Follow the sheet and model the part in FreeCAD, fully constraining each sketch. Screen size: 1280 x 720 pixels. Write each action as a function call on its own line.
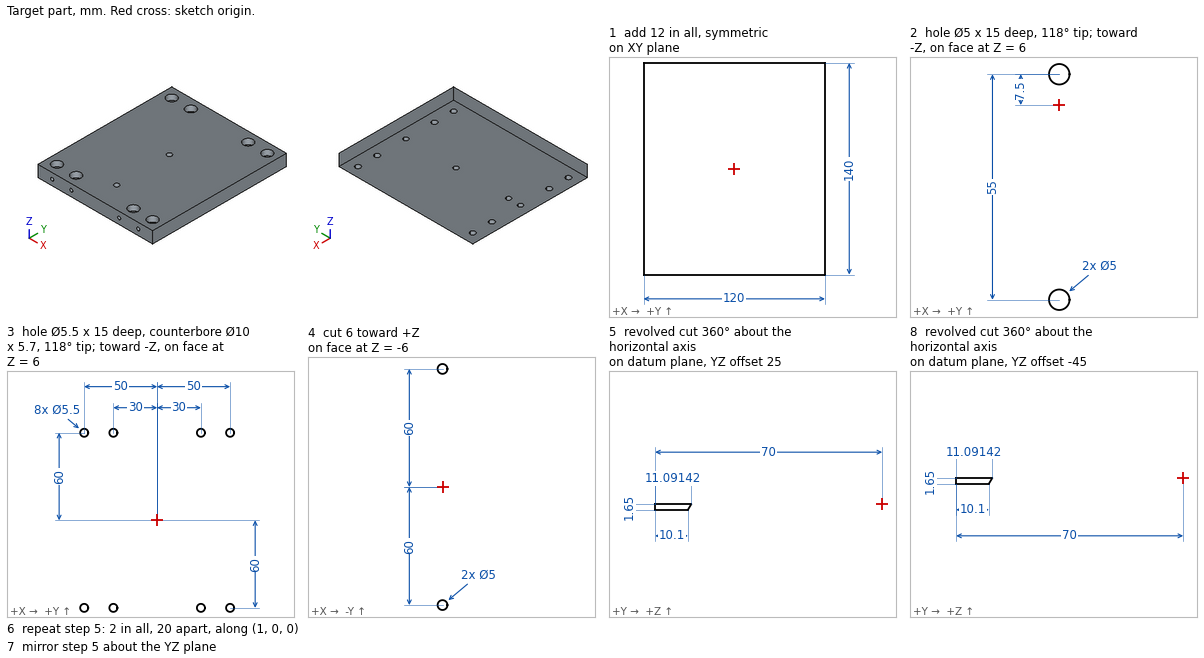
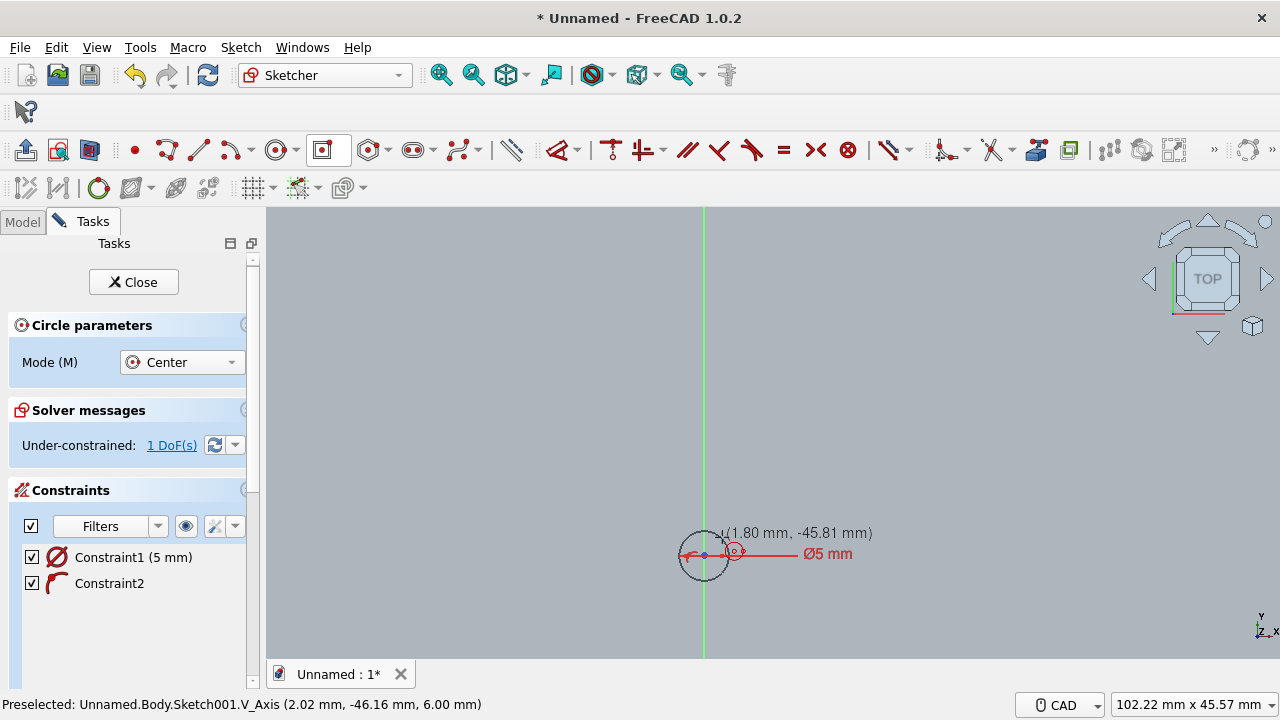
scroll(705, 556, down, 4)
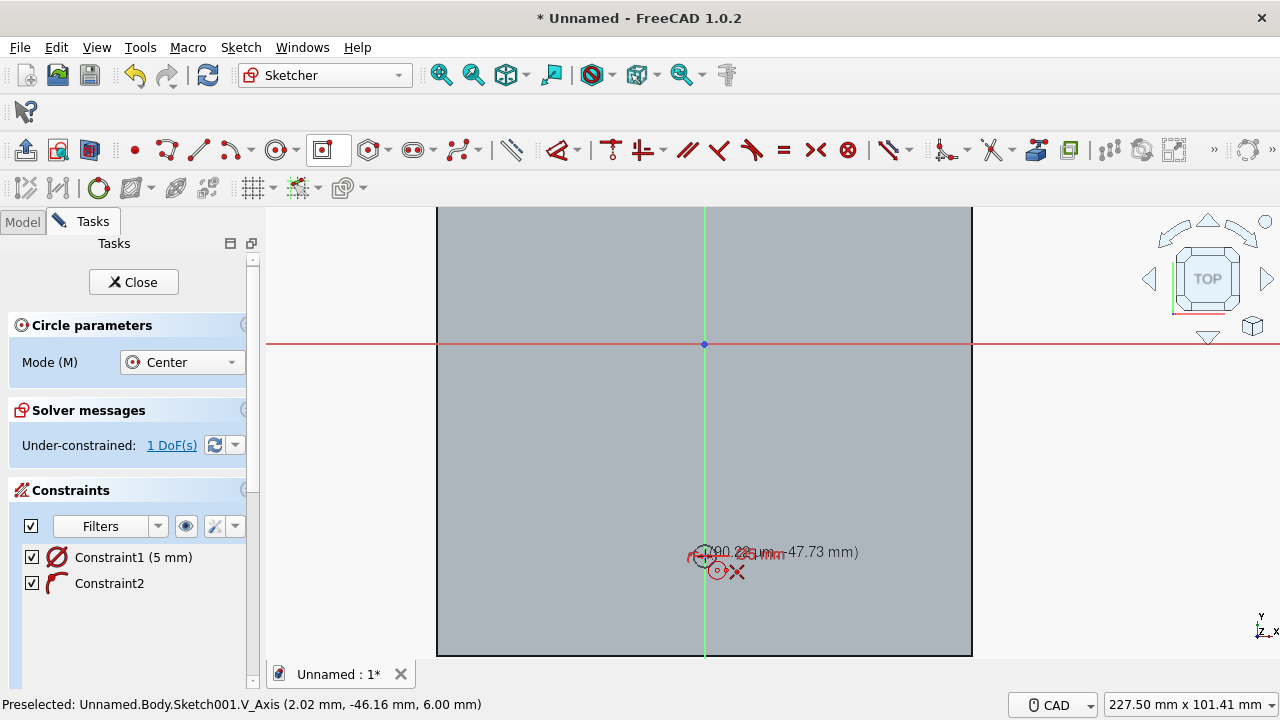
scroll(705, 311, up, 4)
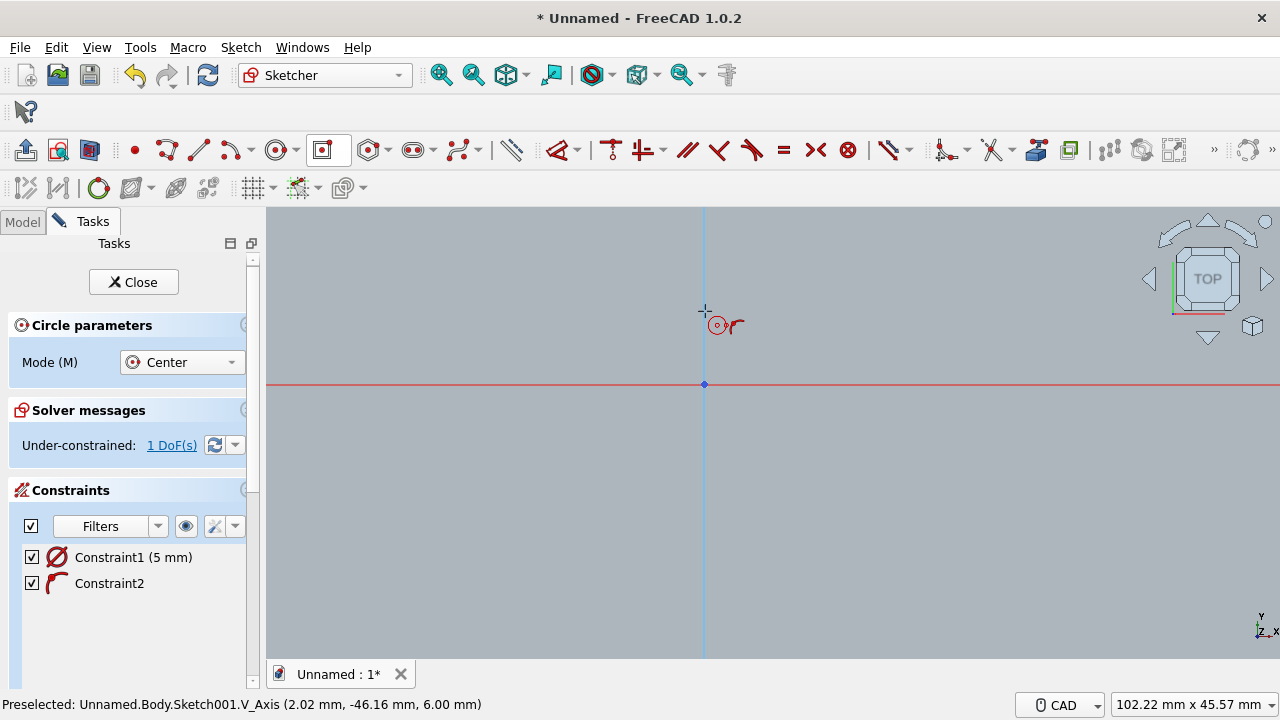
click(704, 310)
move(722, 293)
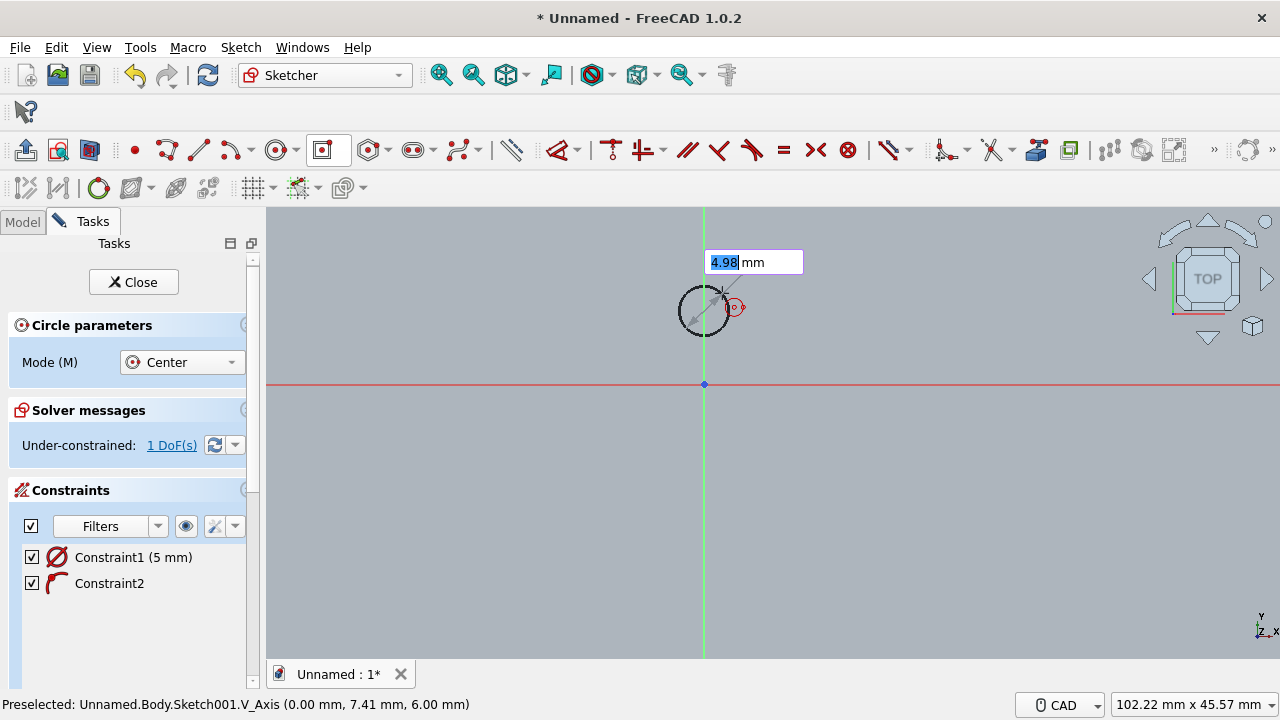
text(5)
key(Return)
key(Escape)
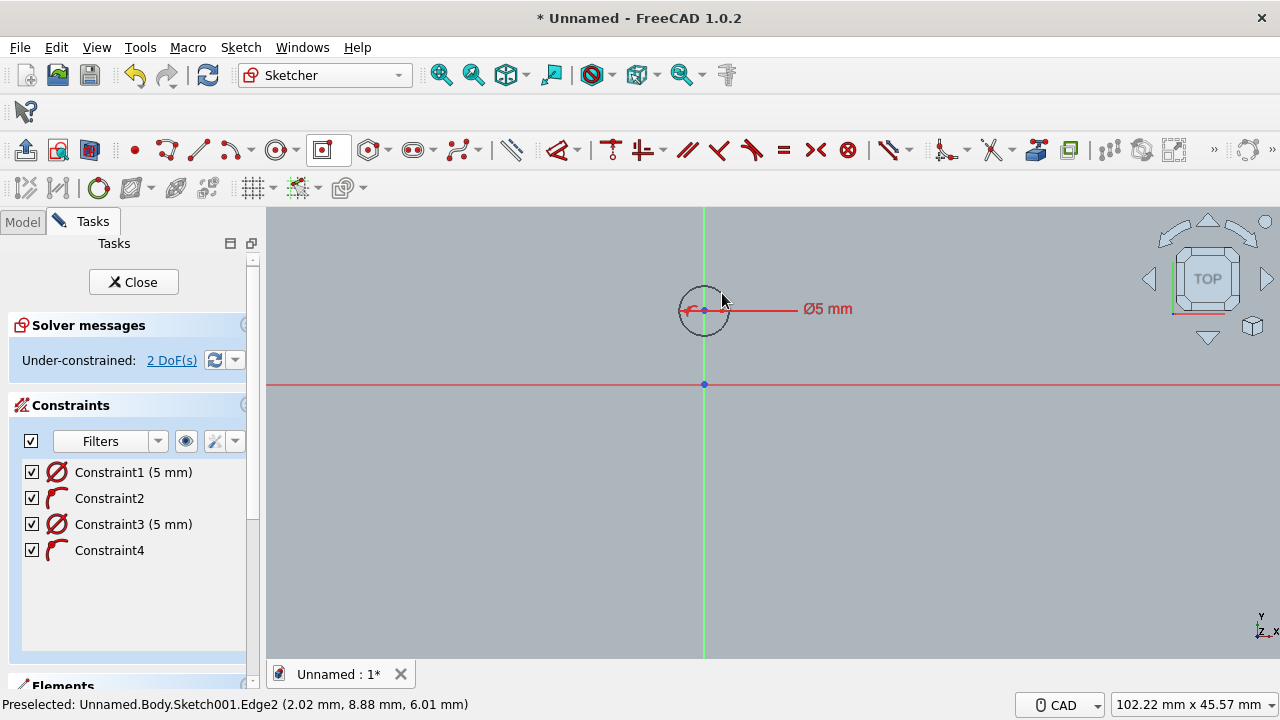
key(d)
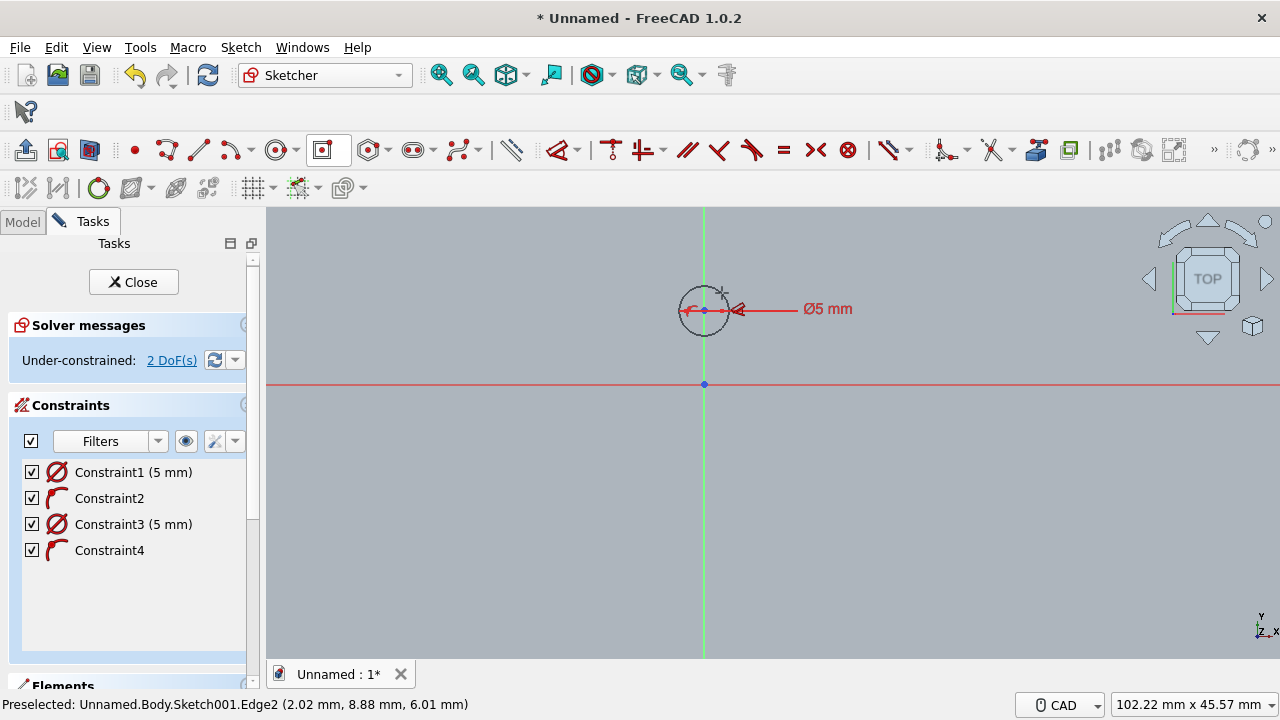
click(704, 311)
click(738, 348)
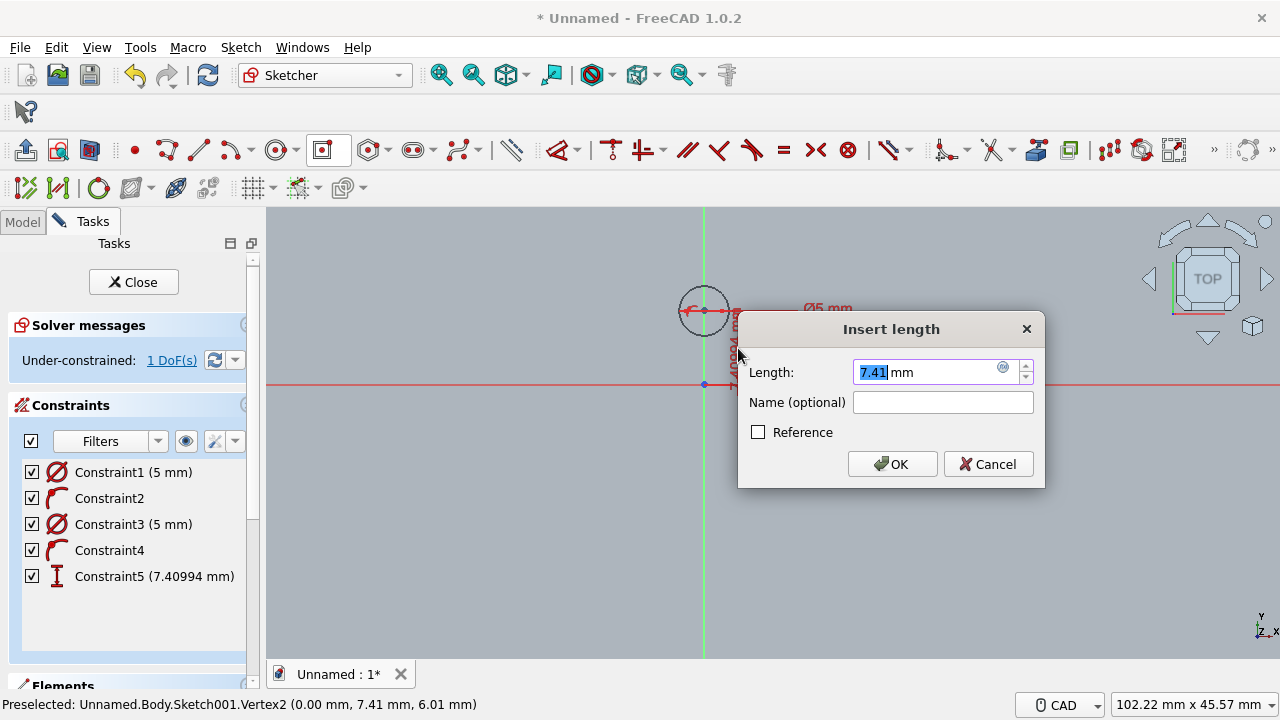
text(7.5)
key(Return)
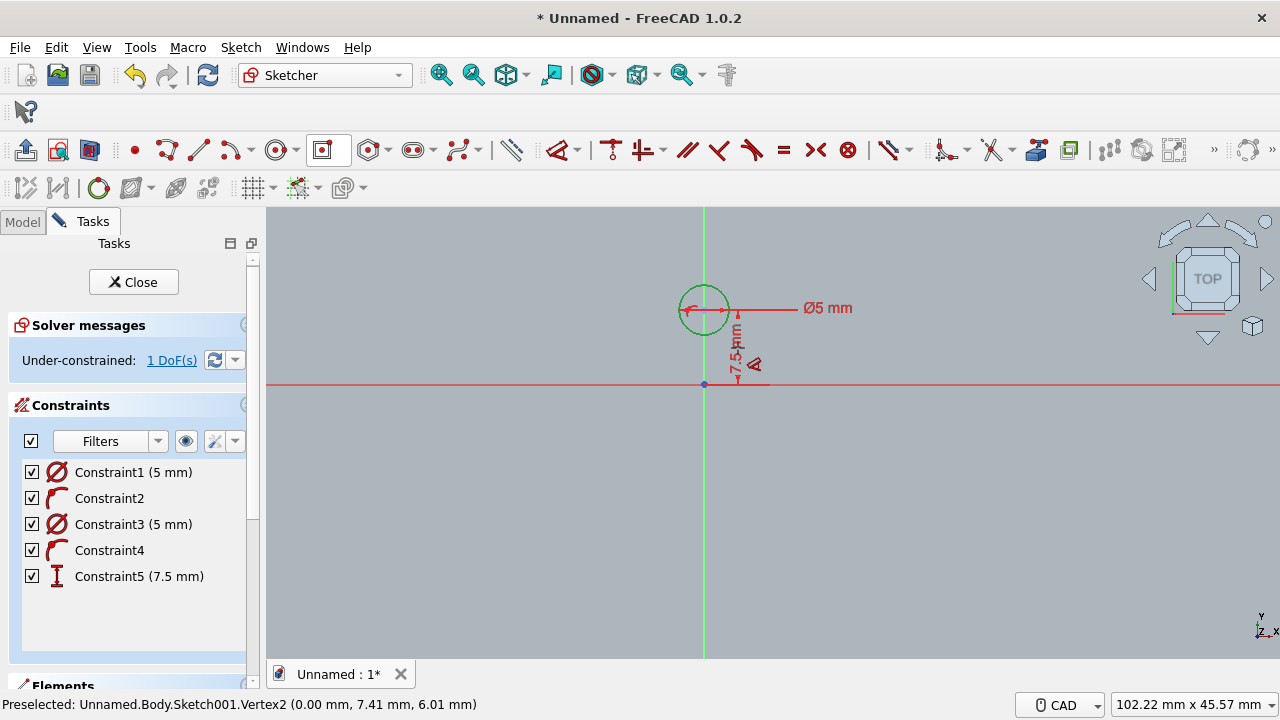
scroll(705, 311, down, 4)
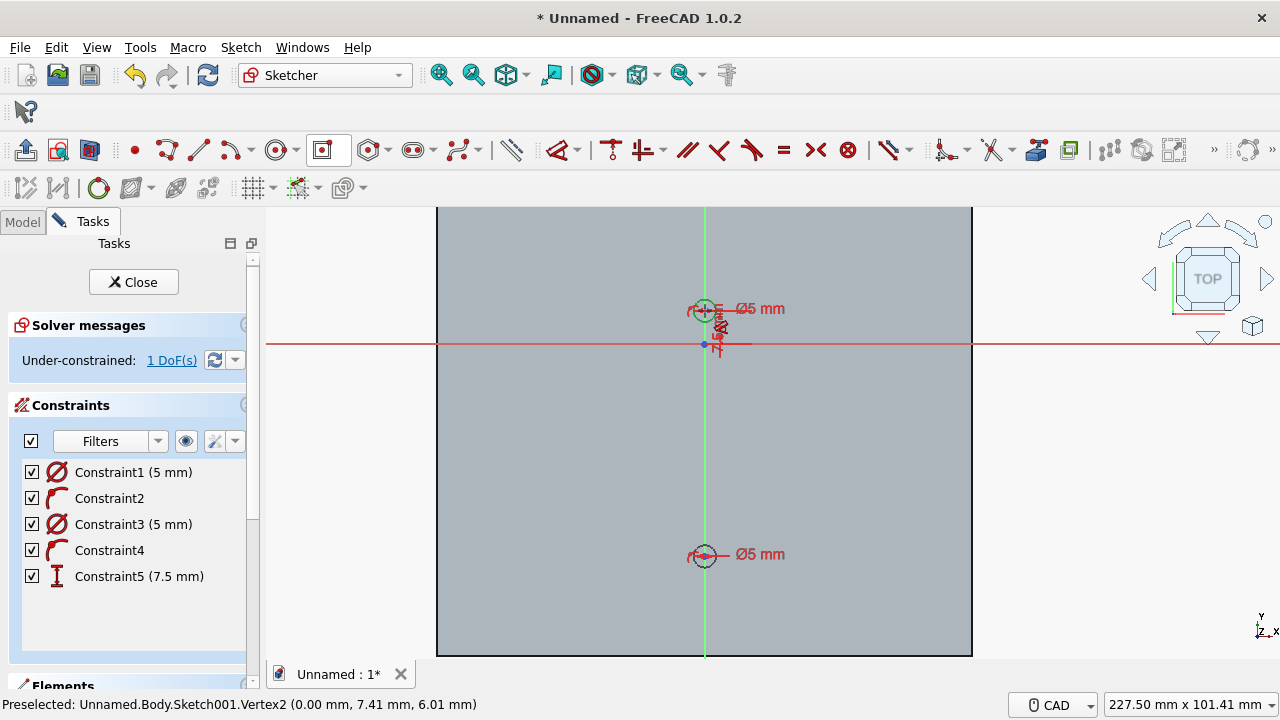
click(705, 556)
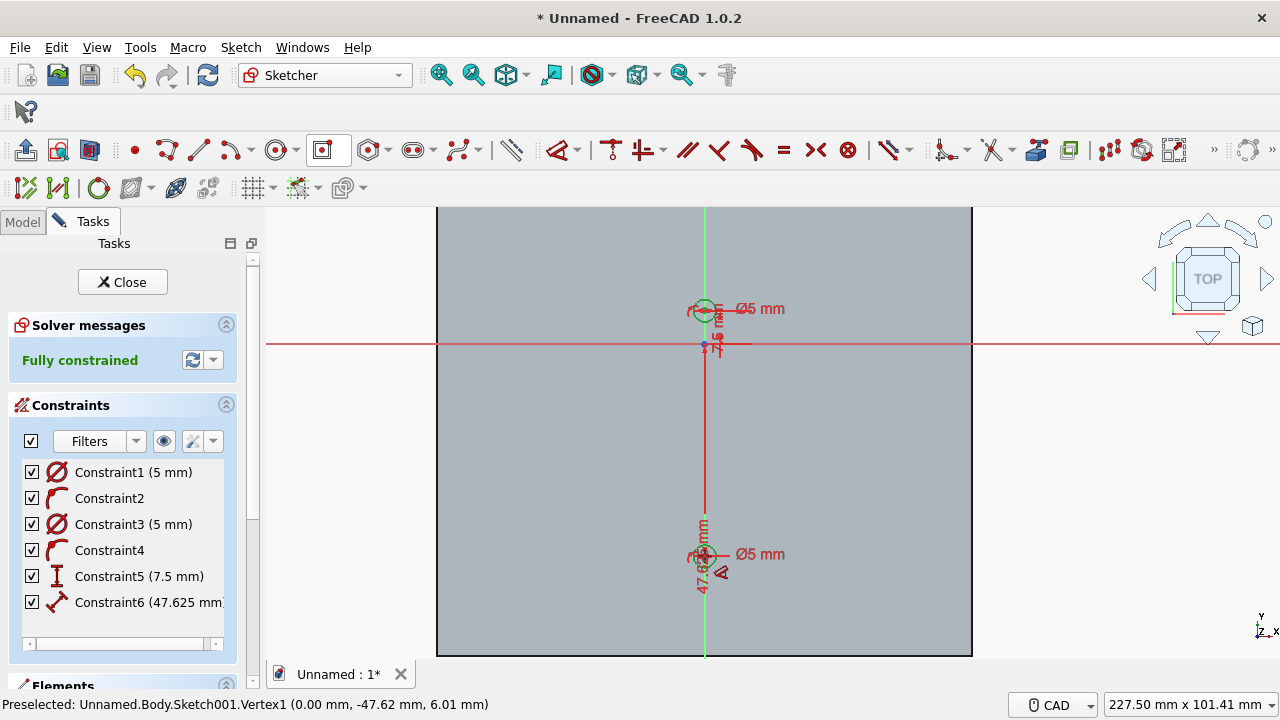
click(705, 311)
click(739, 434)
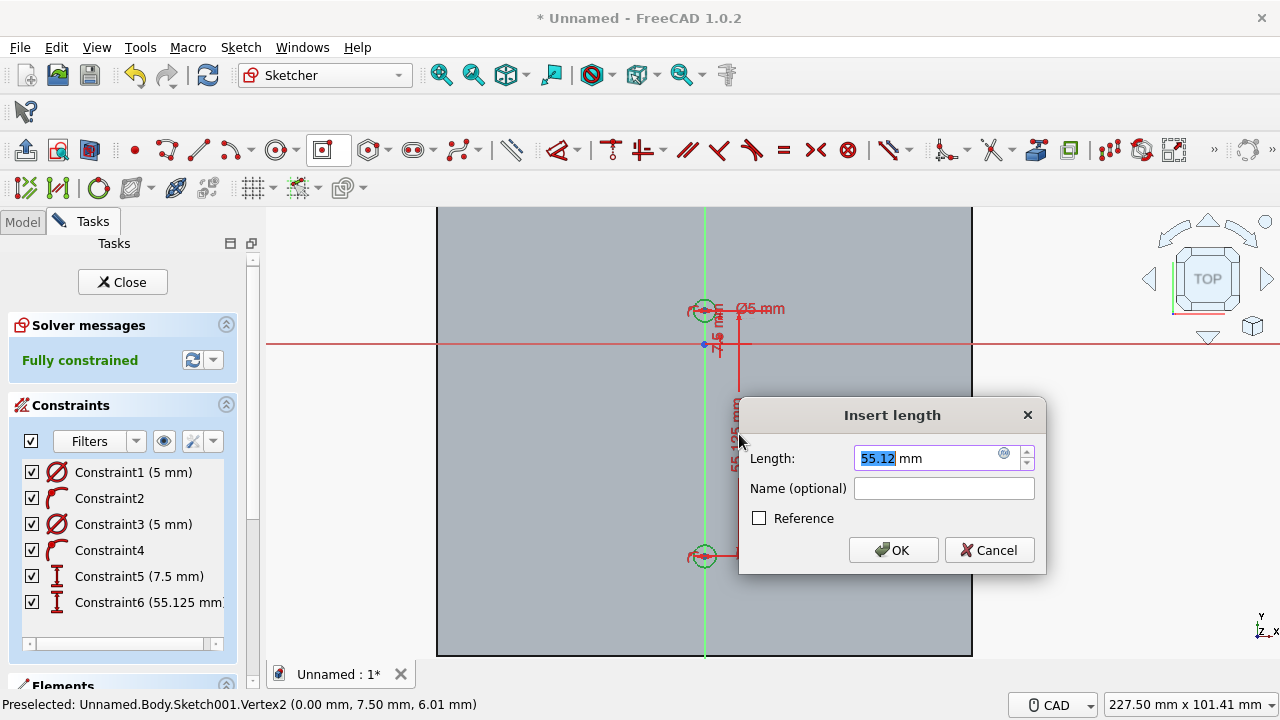
text(55)
key(Return)
key(Escape)